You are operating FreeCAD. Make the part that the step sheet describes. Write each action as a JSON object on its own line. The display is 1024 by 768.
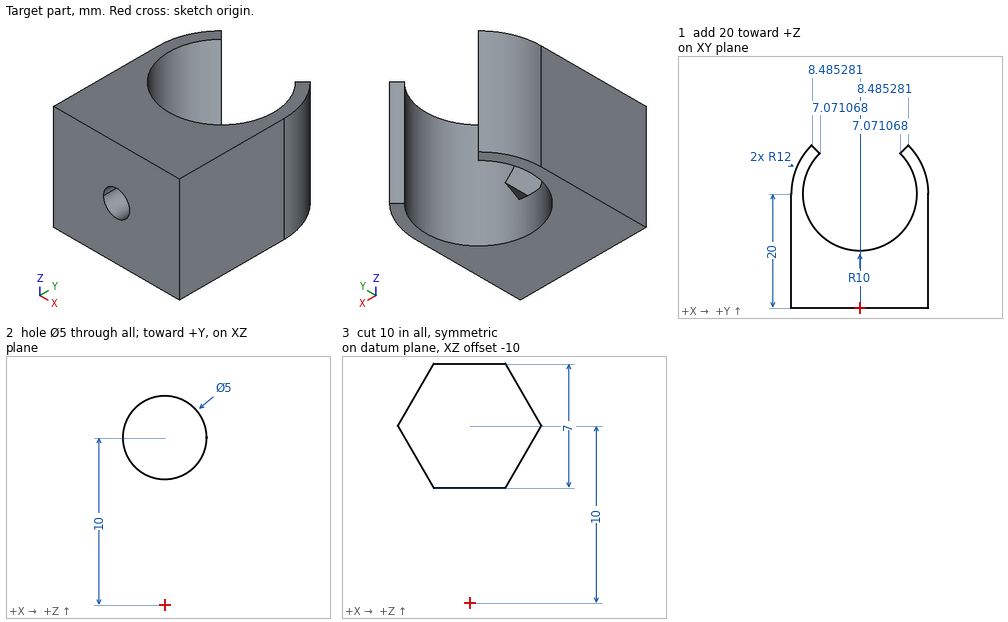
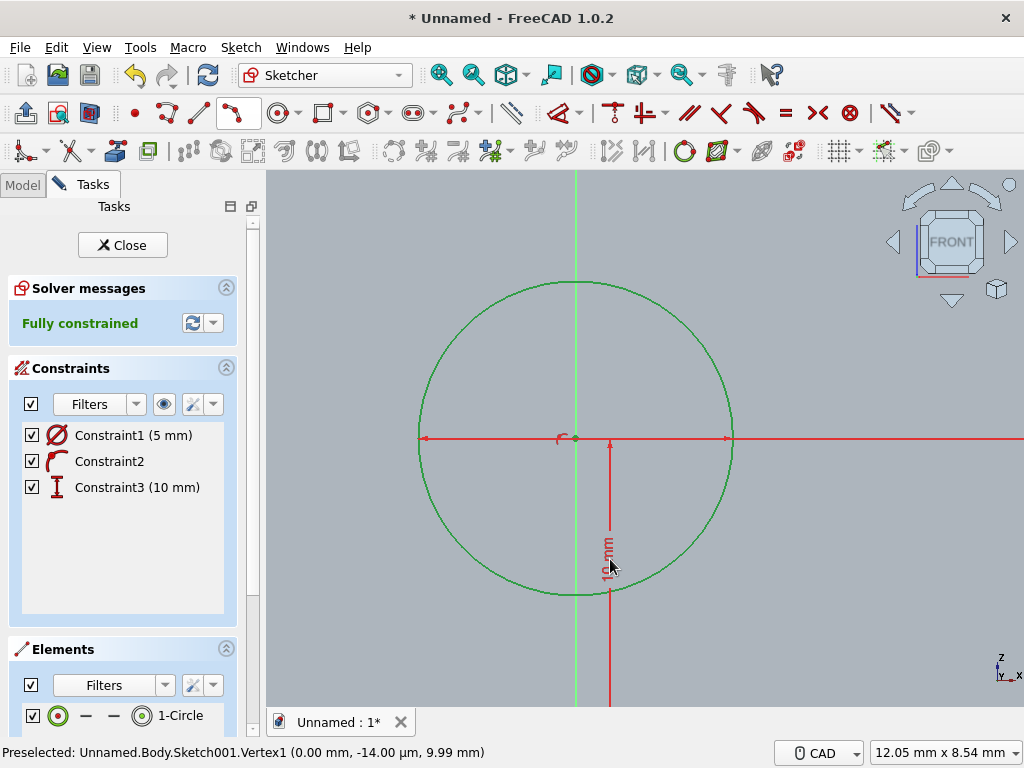
{"action": "left_click", "coordinate": [123, 245]}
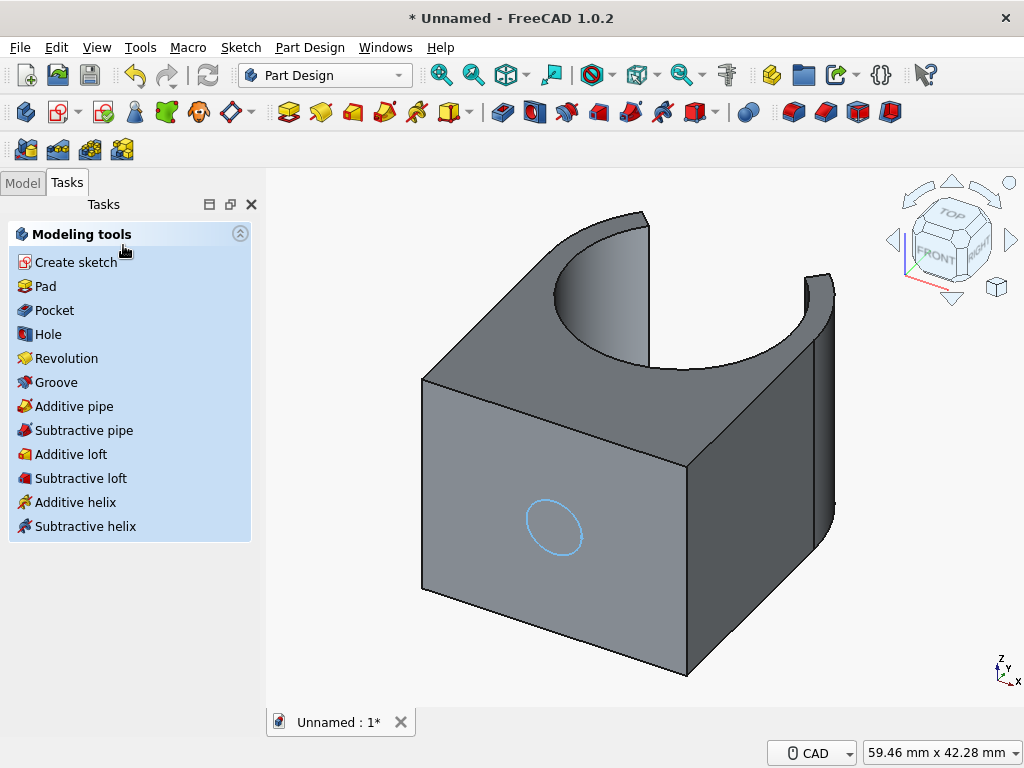
{"action": "left_click", "coordinate": [536, 112]}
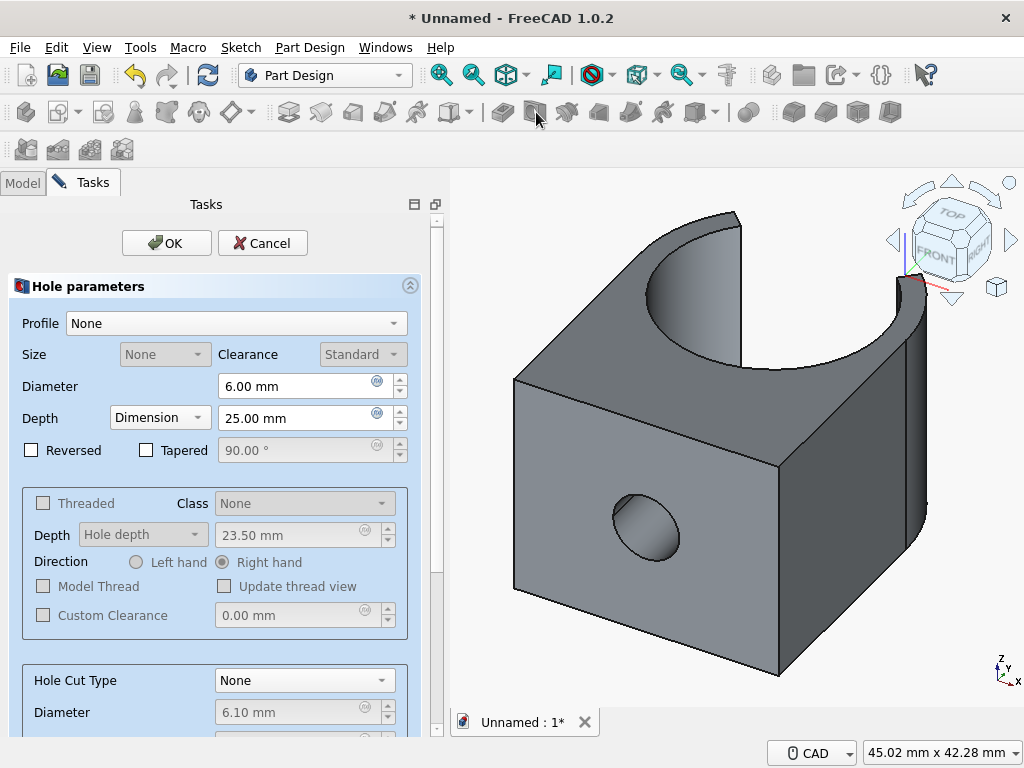
{"action": "triple_click", "coordinate": [305, 386]}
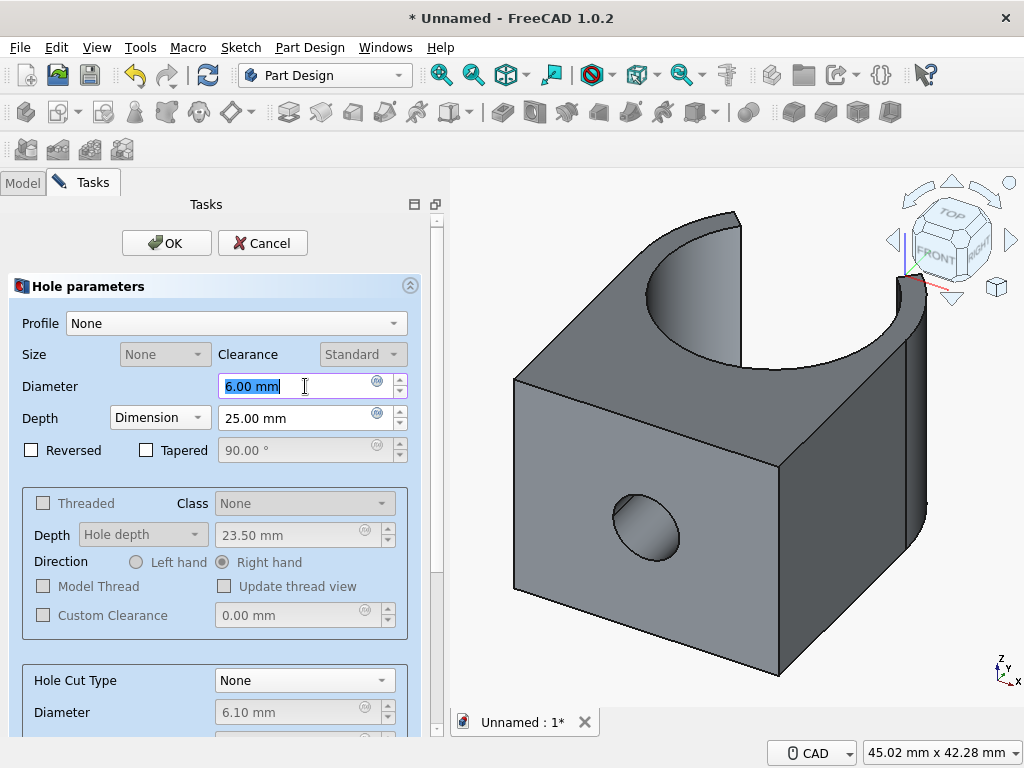
{"action": "type", "text": "5"}
{"action": "key", "text": "Tab"}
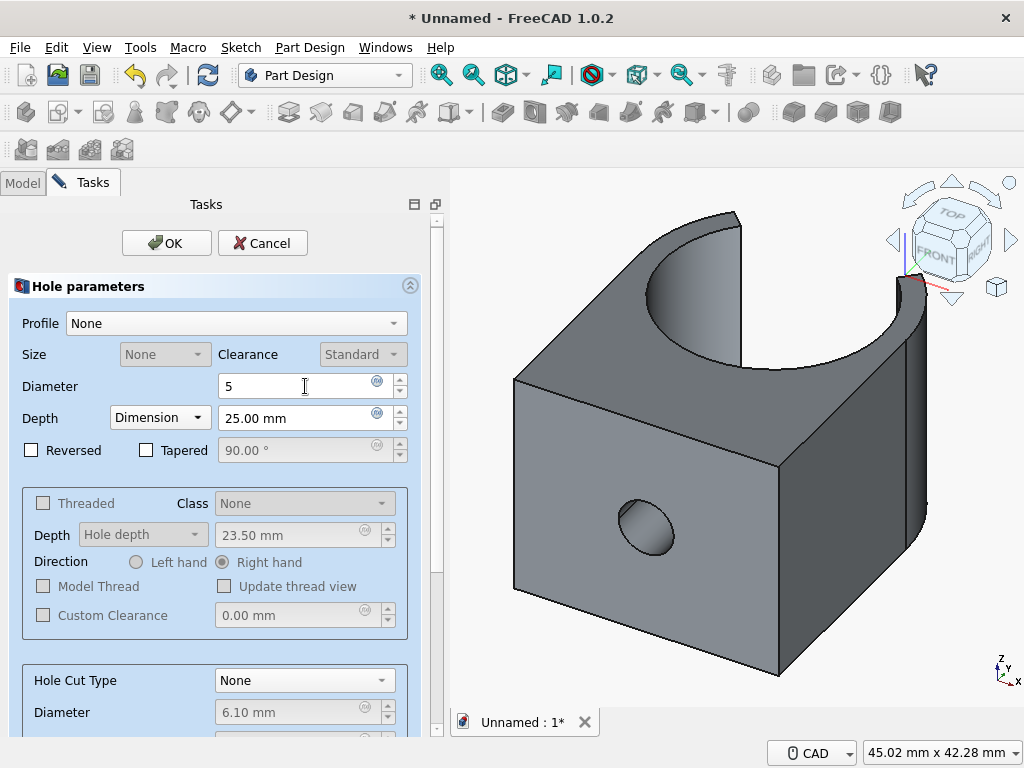
{"action": "left_click", "coordinate": [161, 418]}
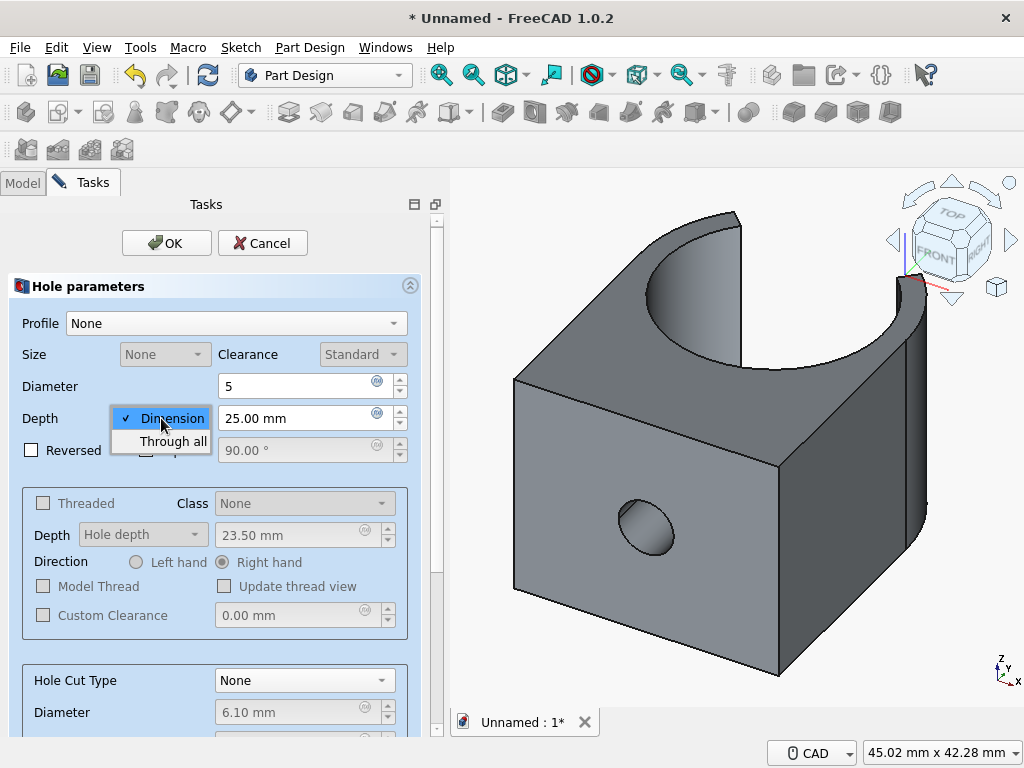
{"action": "left_click", "coordinate": [160, 442]}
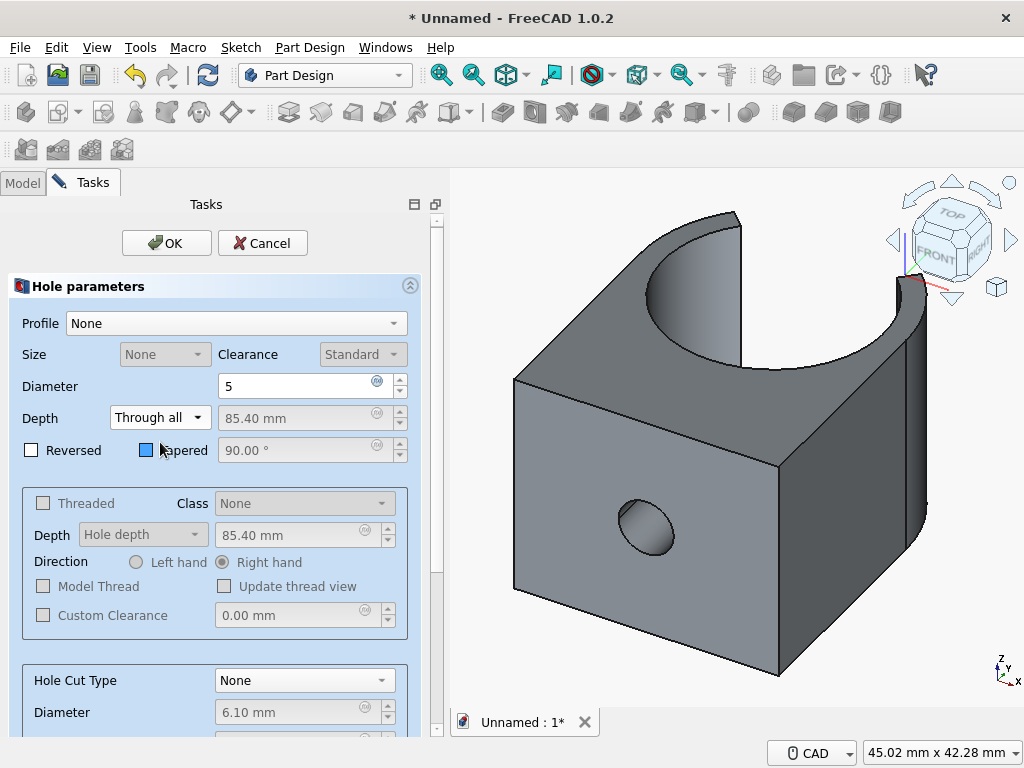
{"action": "left_click", "coordinate": [167, 243]}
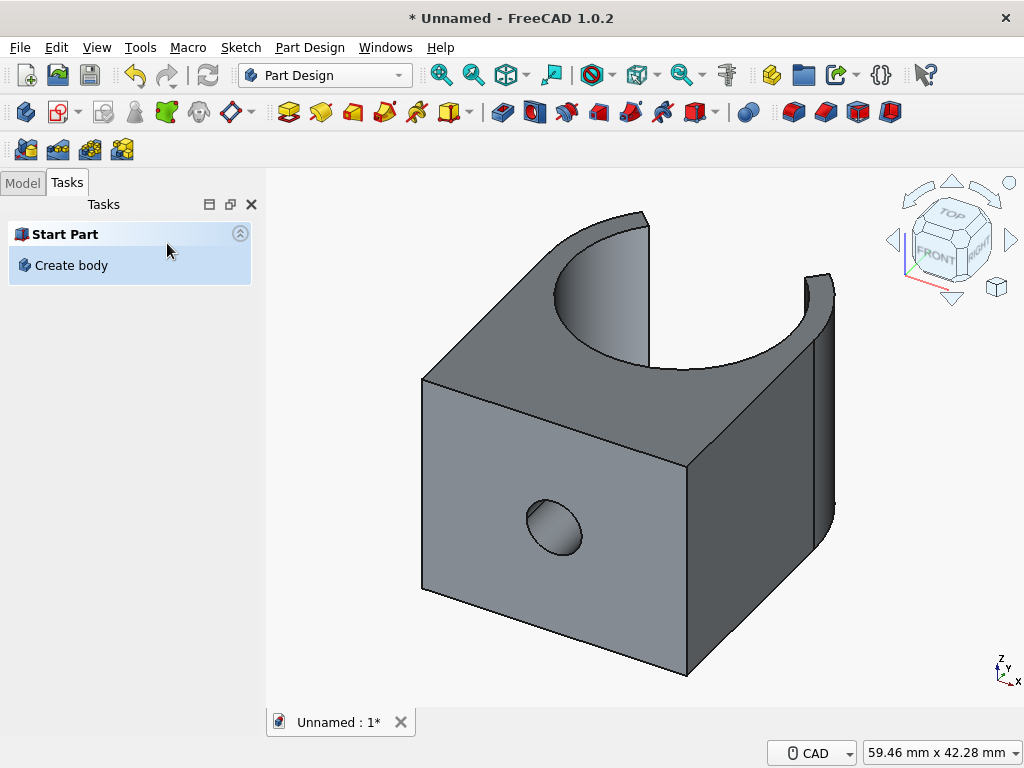
{"action": "left_click", "coordinate": [23, 182]}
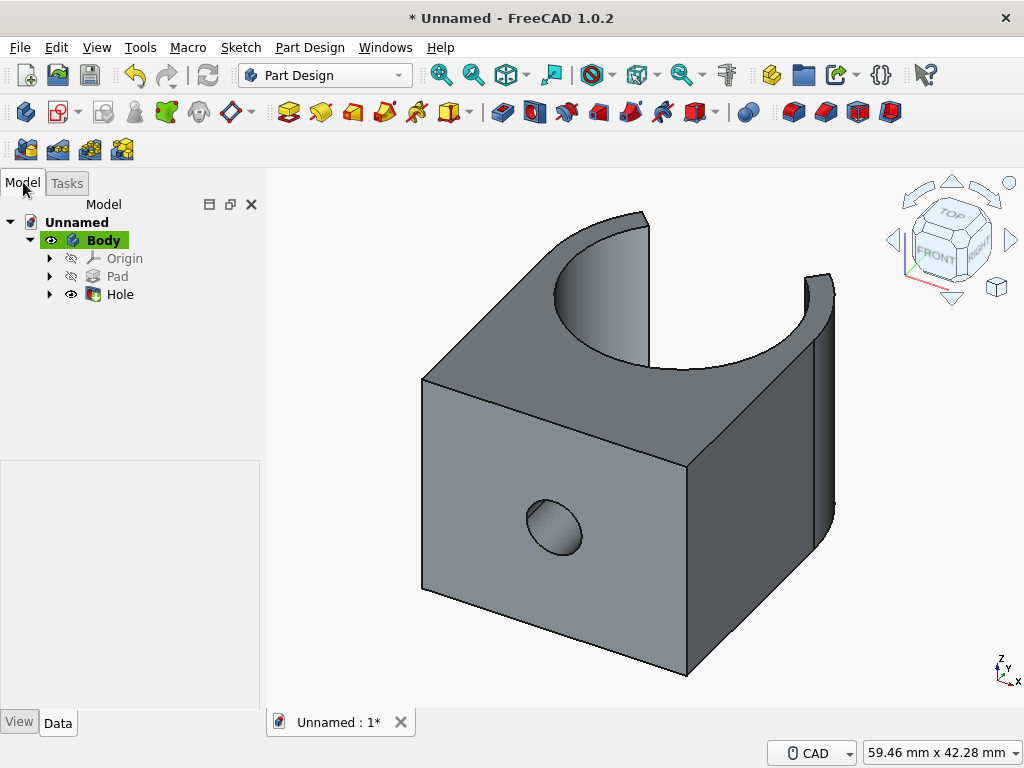
{"action": "left_click", "coordinate": [50, 258]}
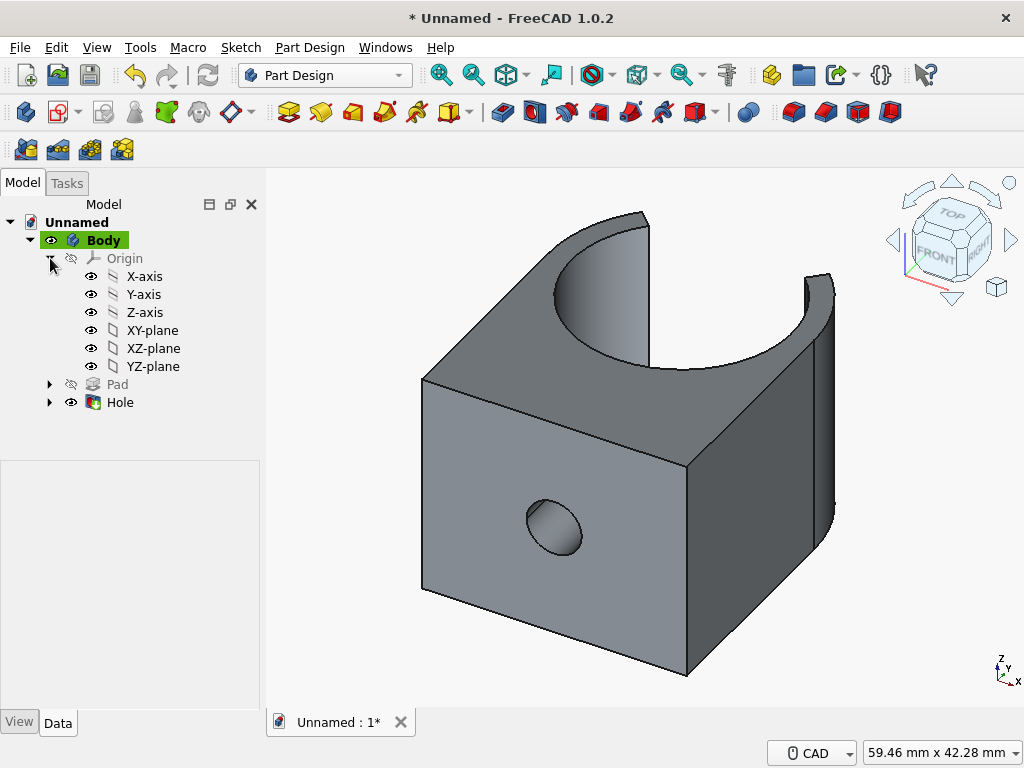
{"action": "left_click", "coordinate": [136, 348]}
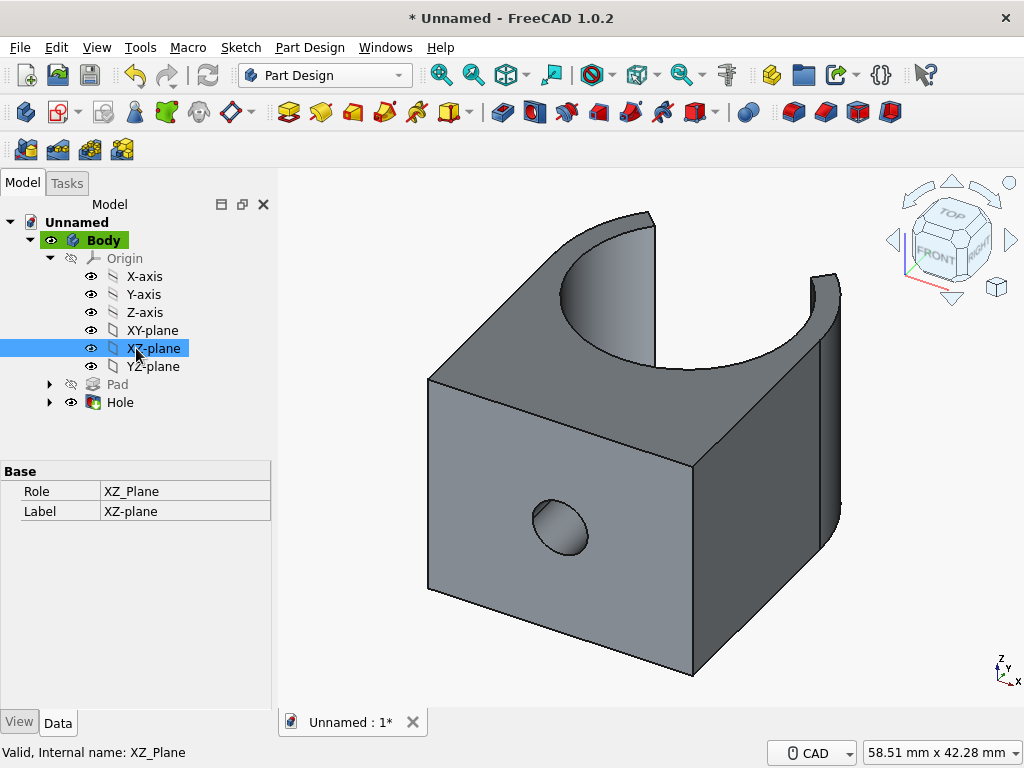
{"action": "left_click", "coordinate": [232, 112]}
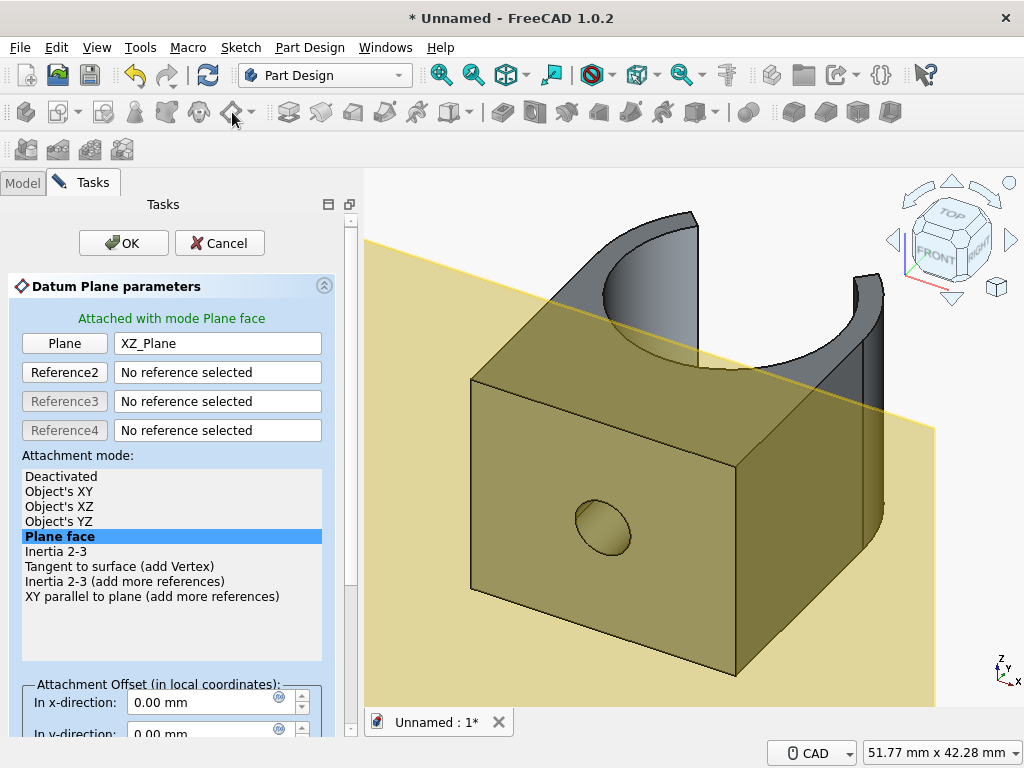
{"action": "scroll", "coordinate": [351, 475], "scroll_direction": "down", "scroll_amount": 2}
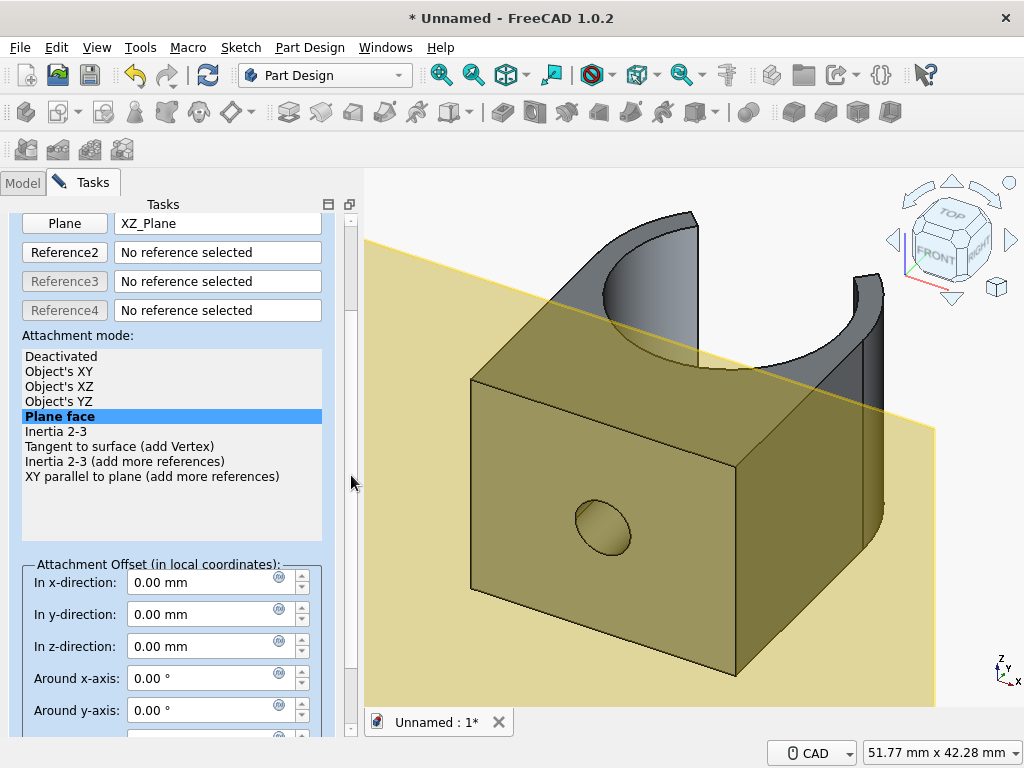
{"action": "triple_click", "coordinate": [210, 646]}